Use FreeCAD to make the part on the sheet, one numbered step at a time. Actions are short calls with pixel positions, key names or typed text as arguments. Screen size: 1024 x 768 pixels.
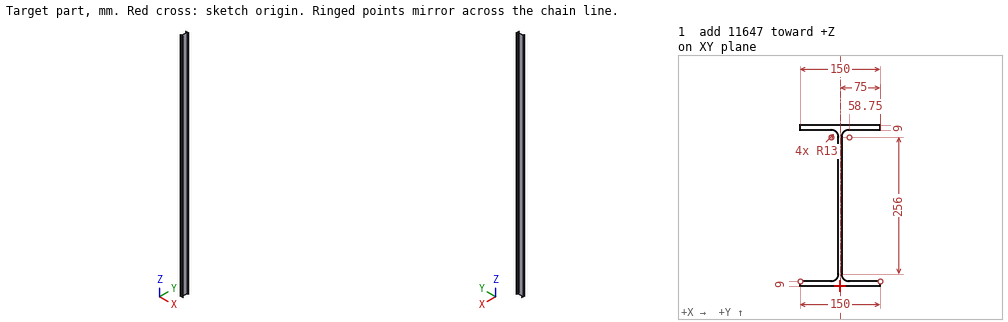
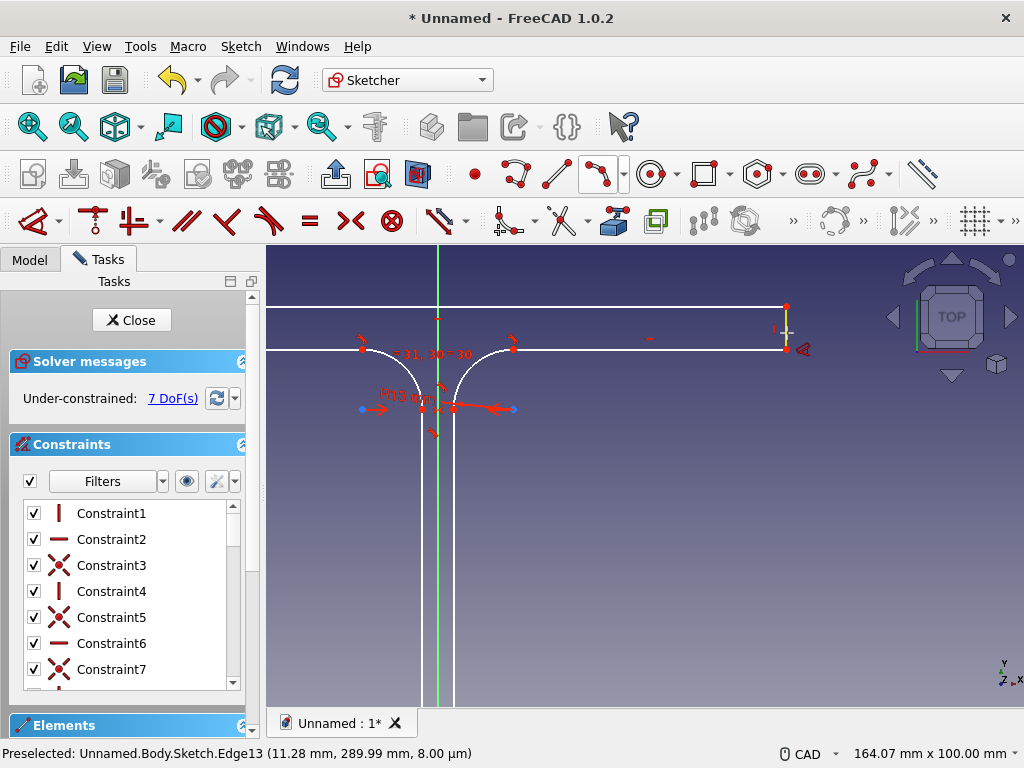
click(786, 332)
click(820, 328)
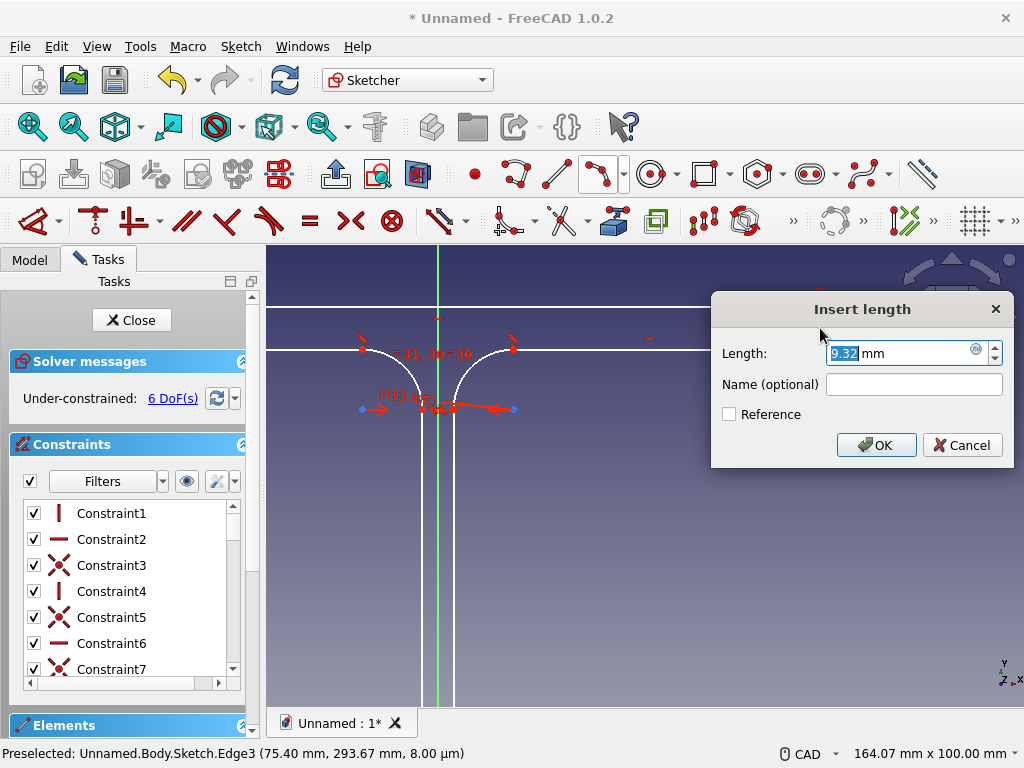
text(9)
key(Return)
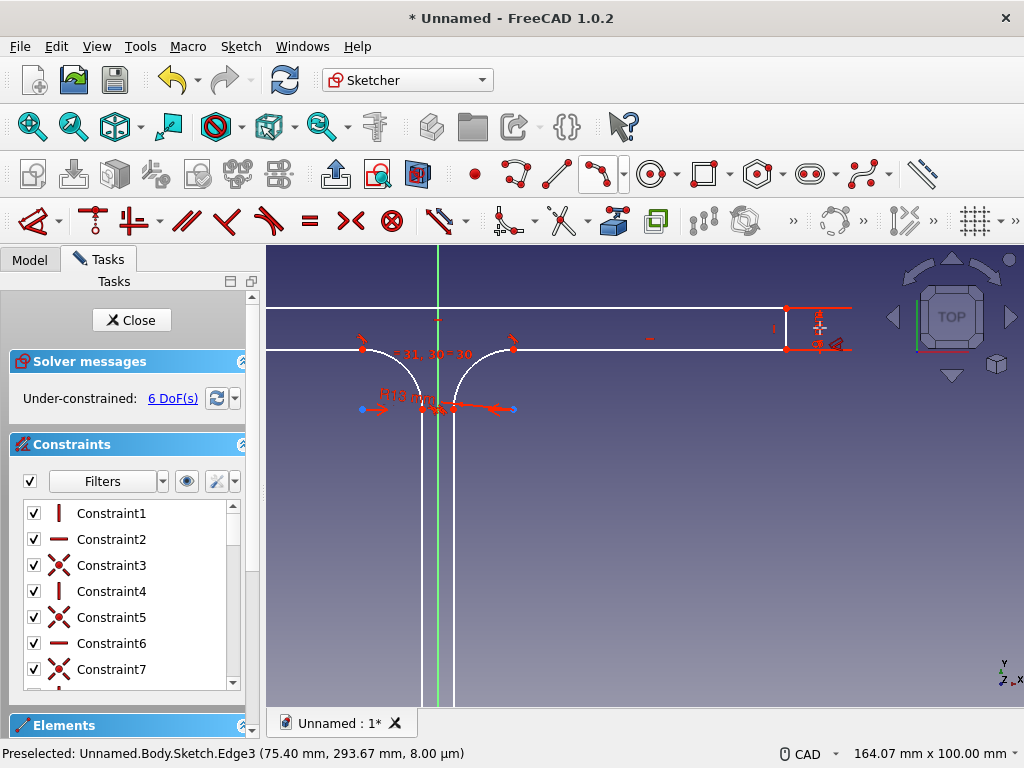
scroll(612, 344, down, 8)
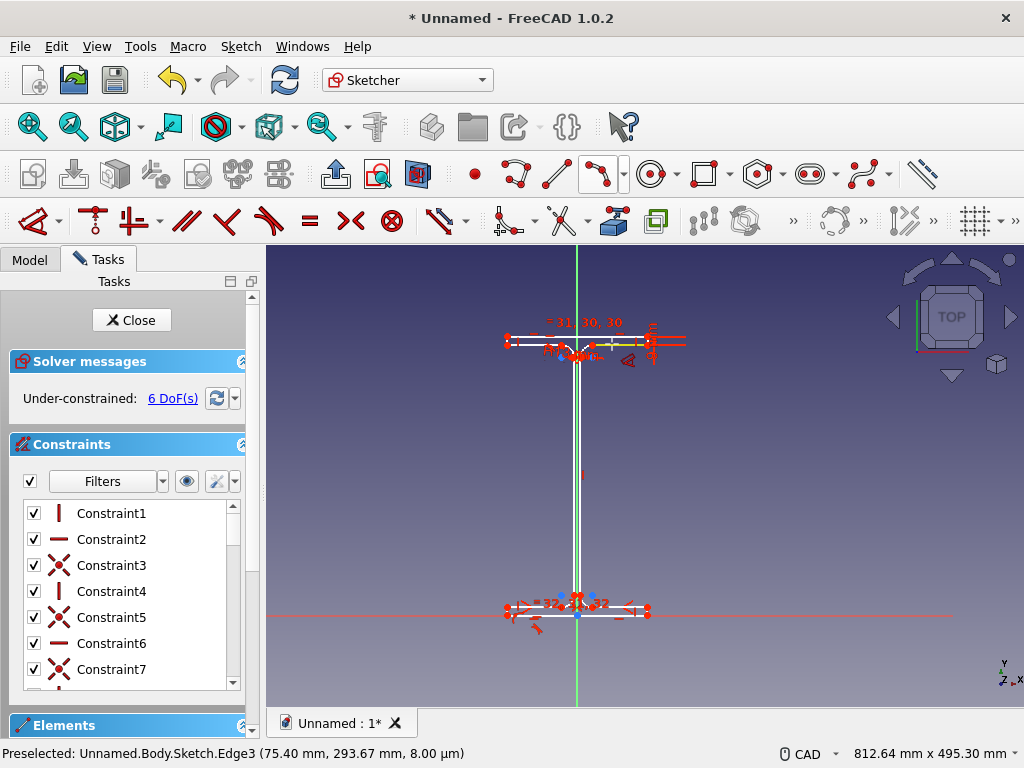
scroll(507, 610, up, 9)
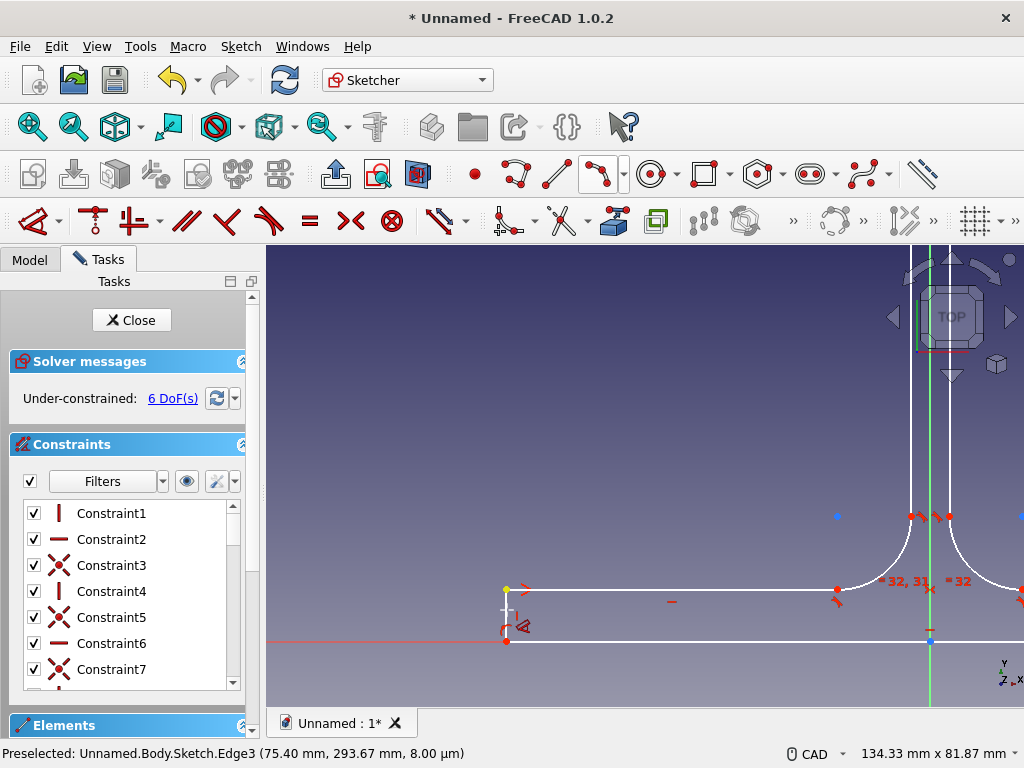
click(506, 605)
click(472, 616)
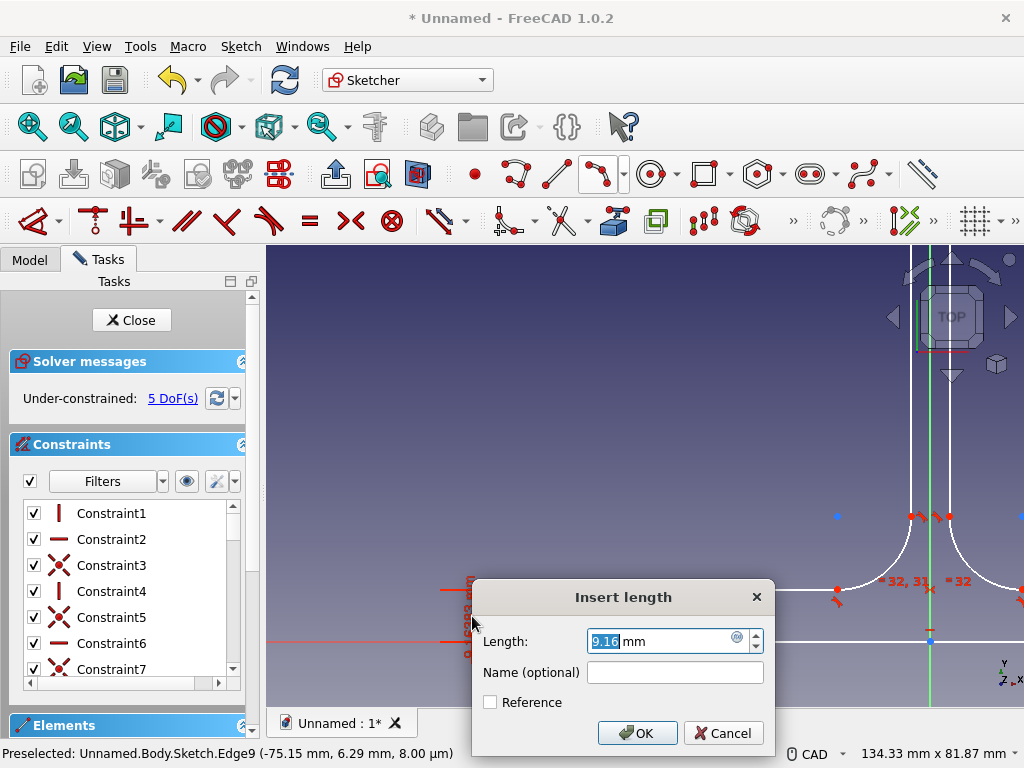
text(9)
key(Return)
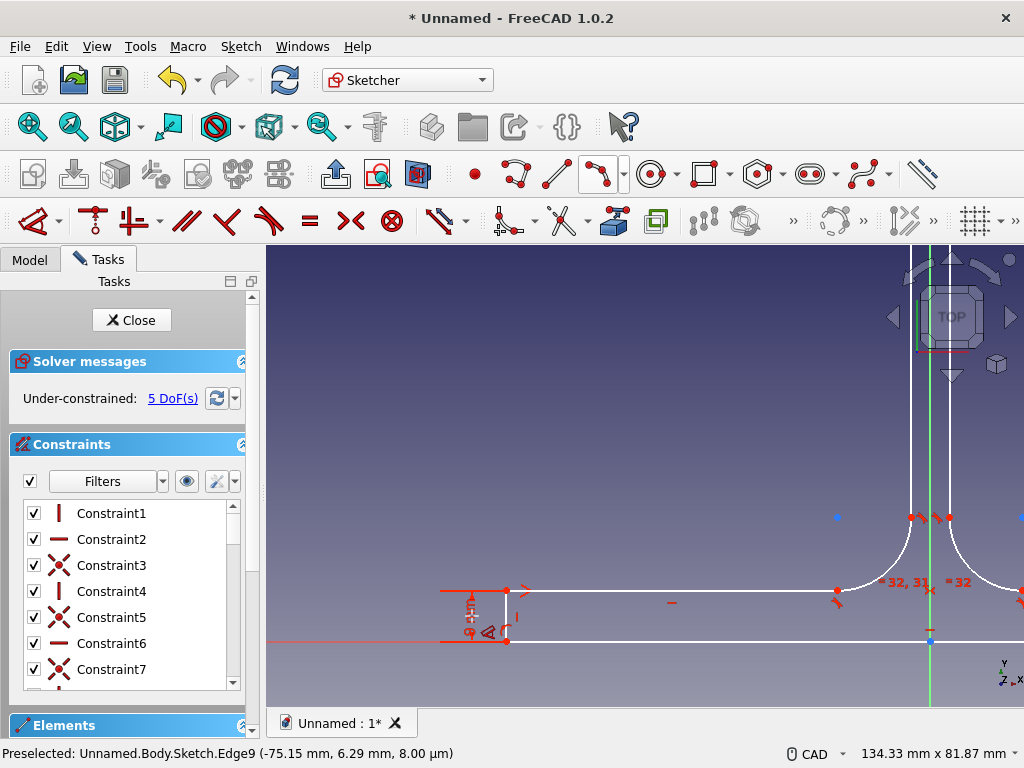
scroll(506, 611, down, 9)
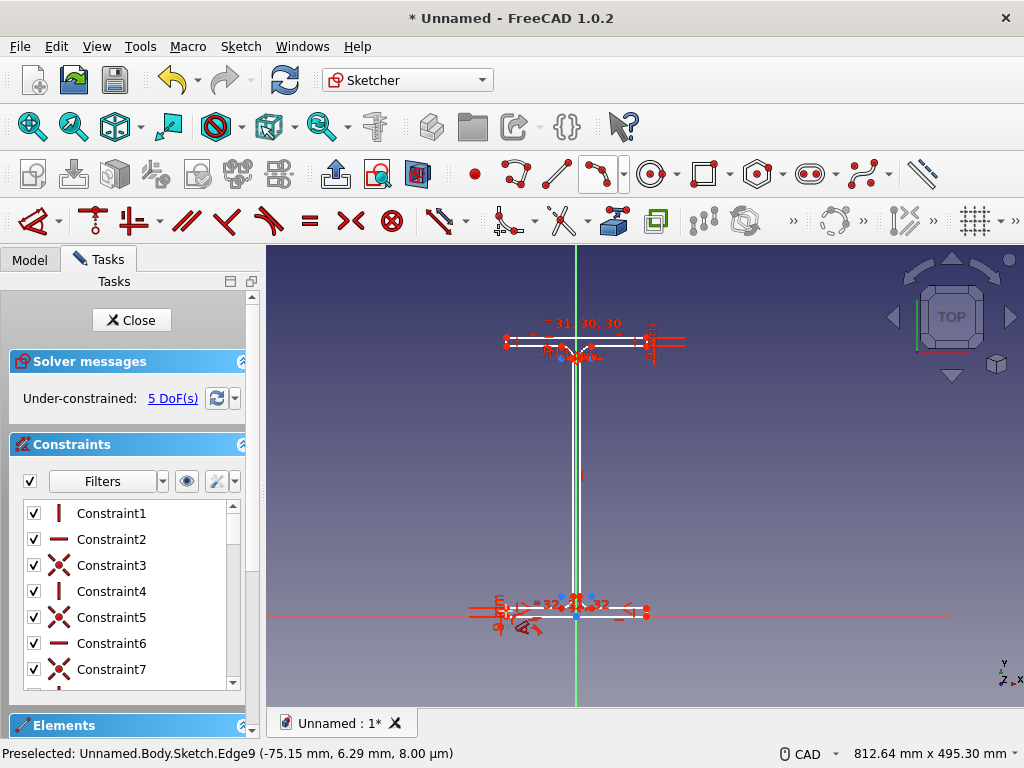
scroll(580, 525, up, 8)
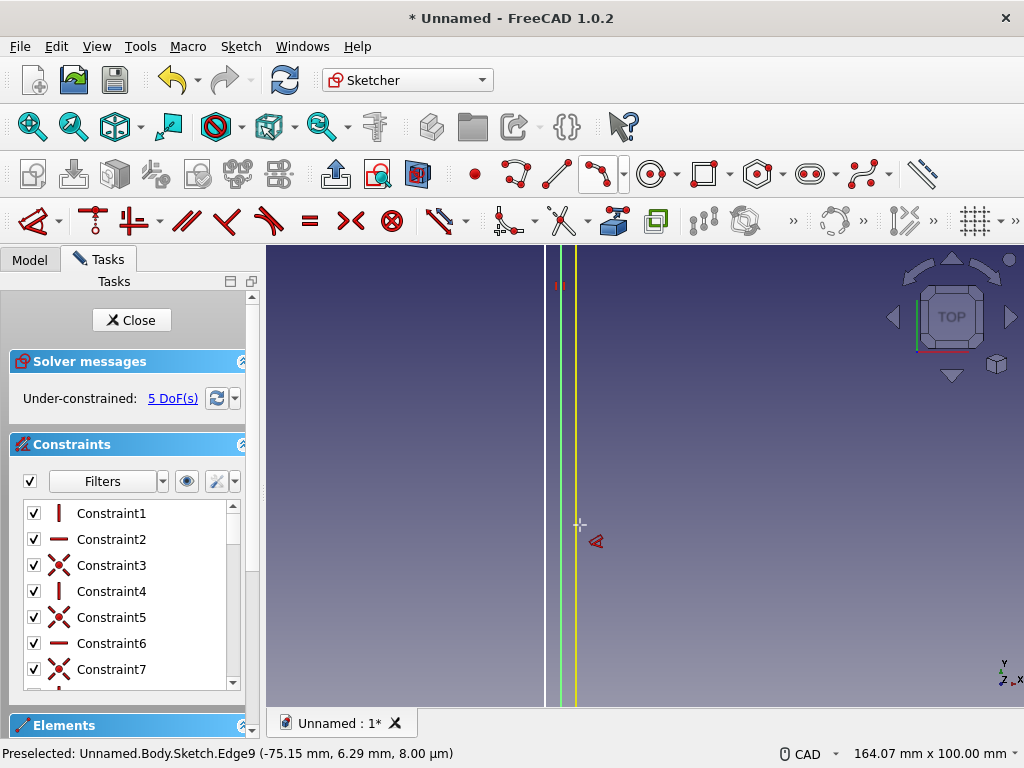
click(576, 522)
click(610, 476)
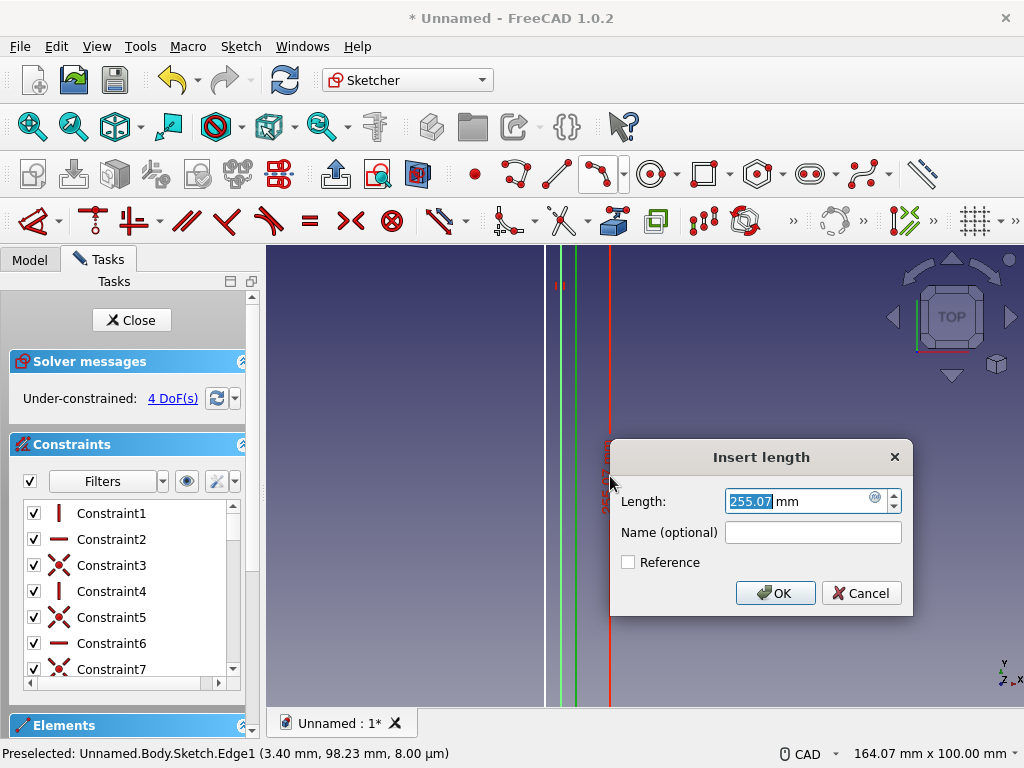
text(256)
key(Return)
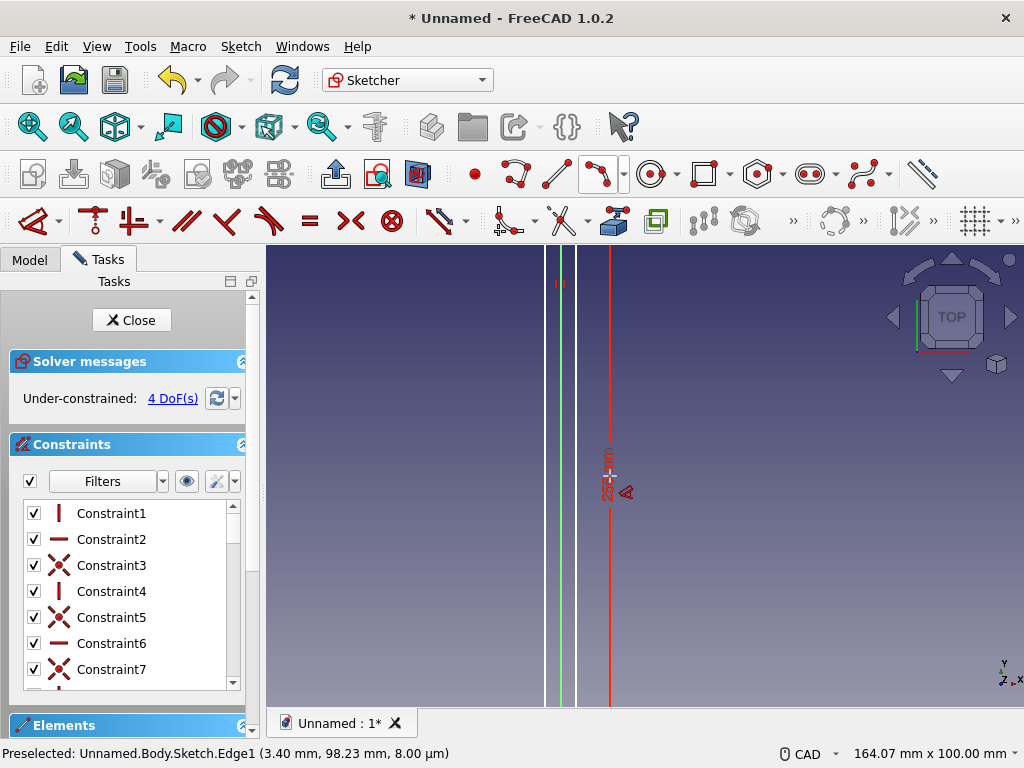
scroll(581, 525, down, 8)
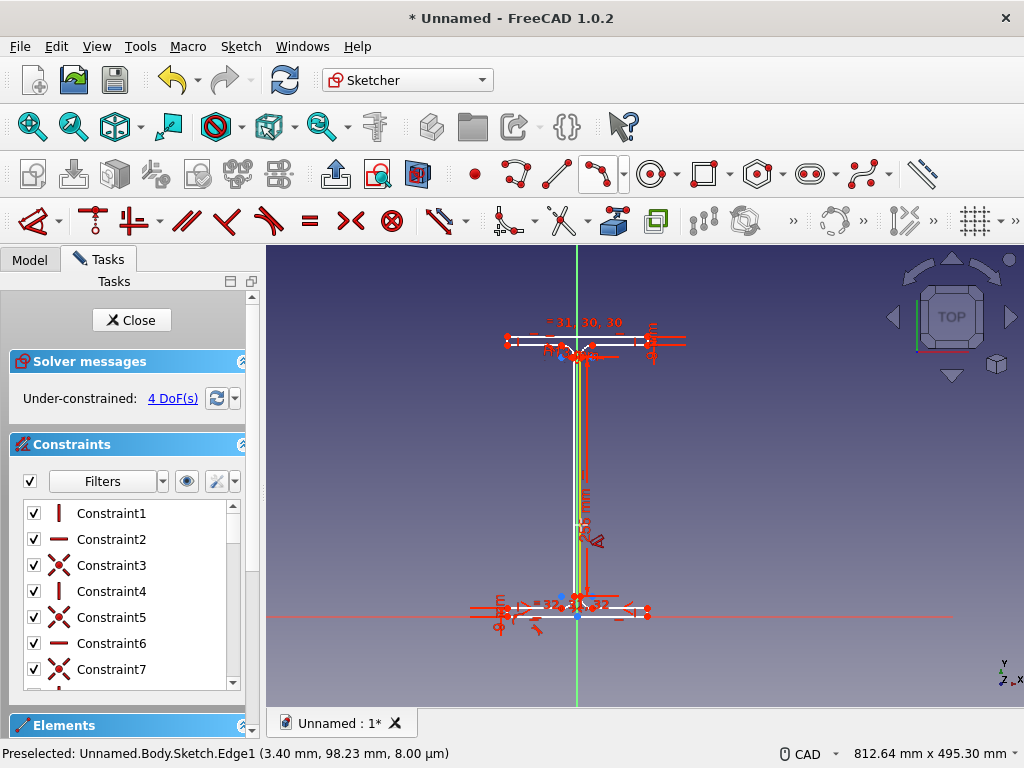
scroll(605, 337, up, 3)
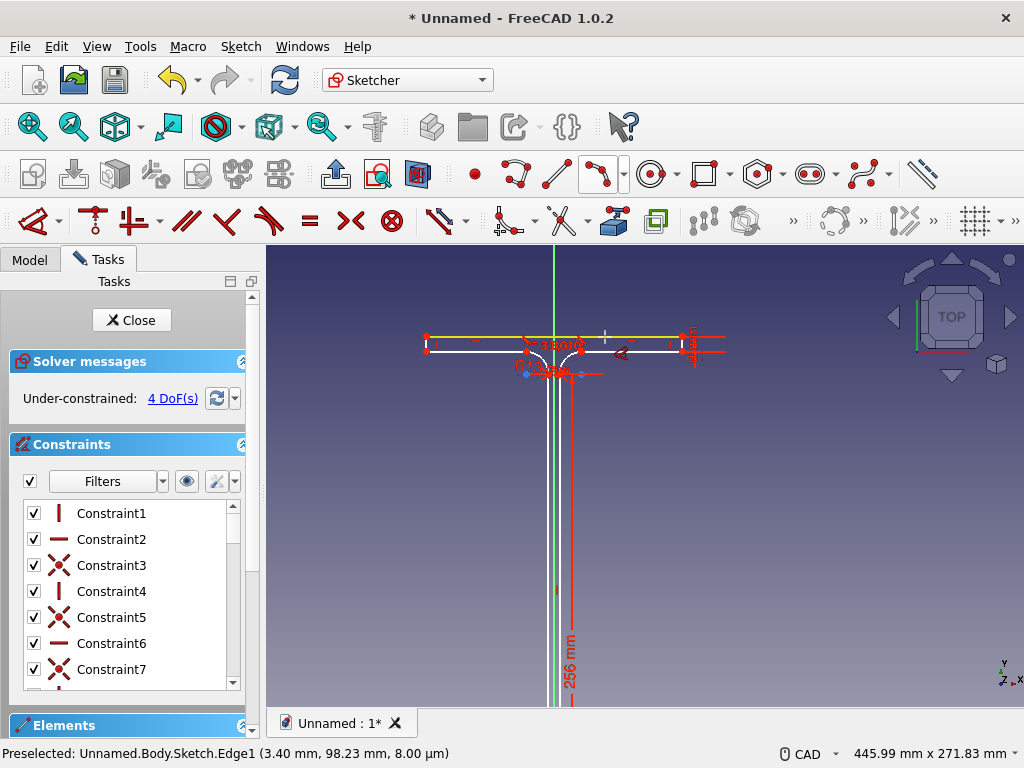
click(605, 337)
click(495, 303)